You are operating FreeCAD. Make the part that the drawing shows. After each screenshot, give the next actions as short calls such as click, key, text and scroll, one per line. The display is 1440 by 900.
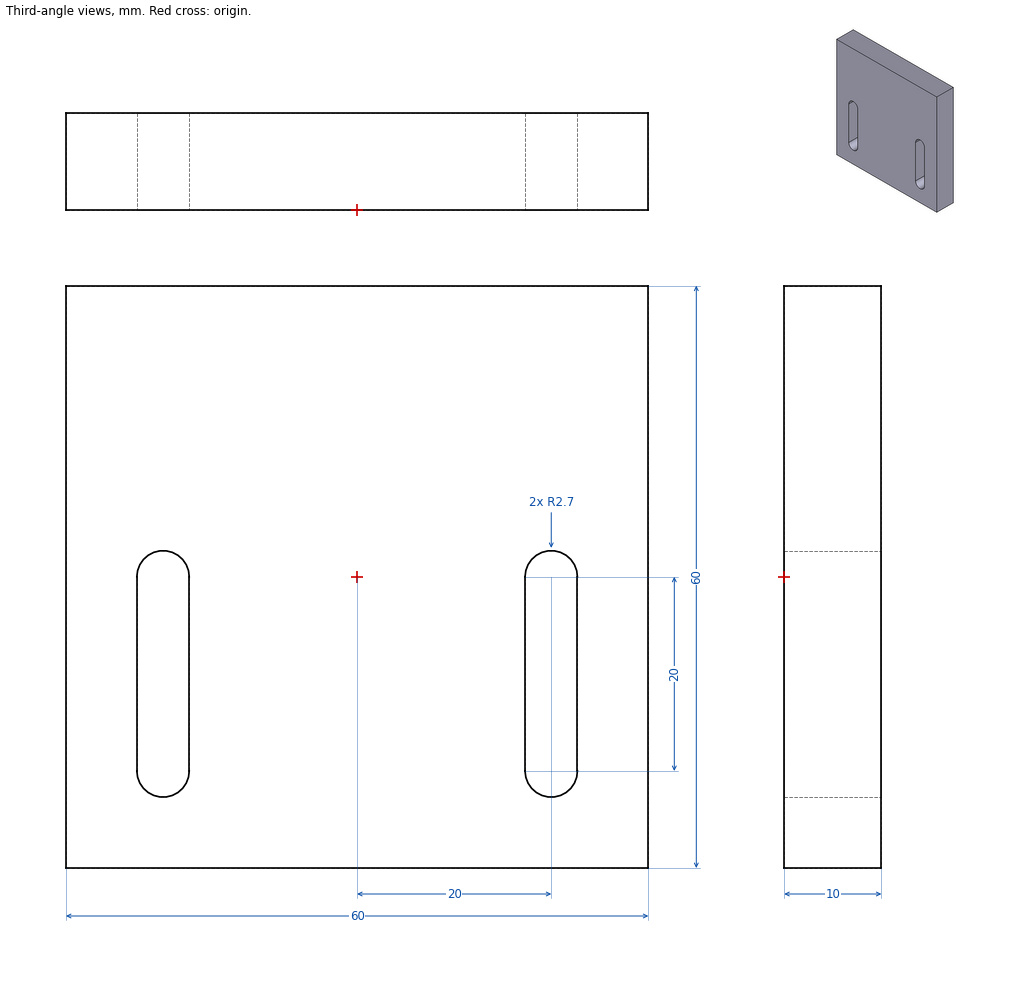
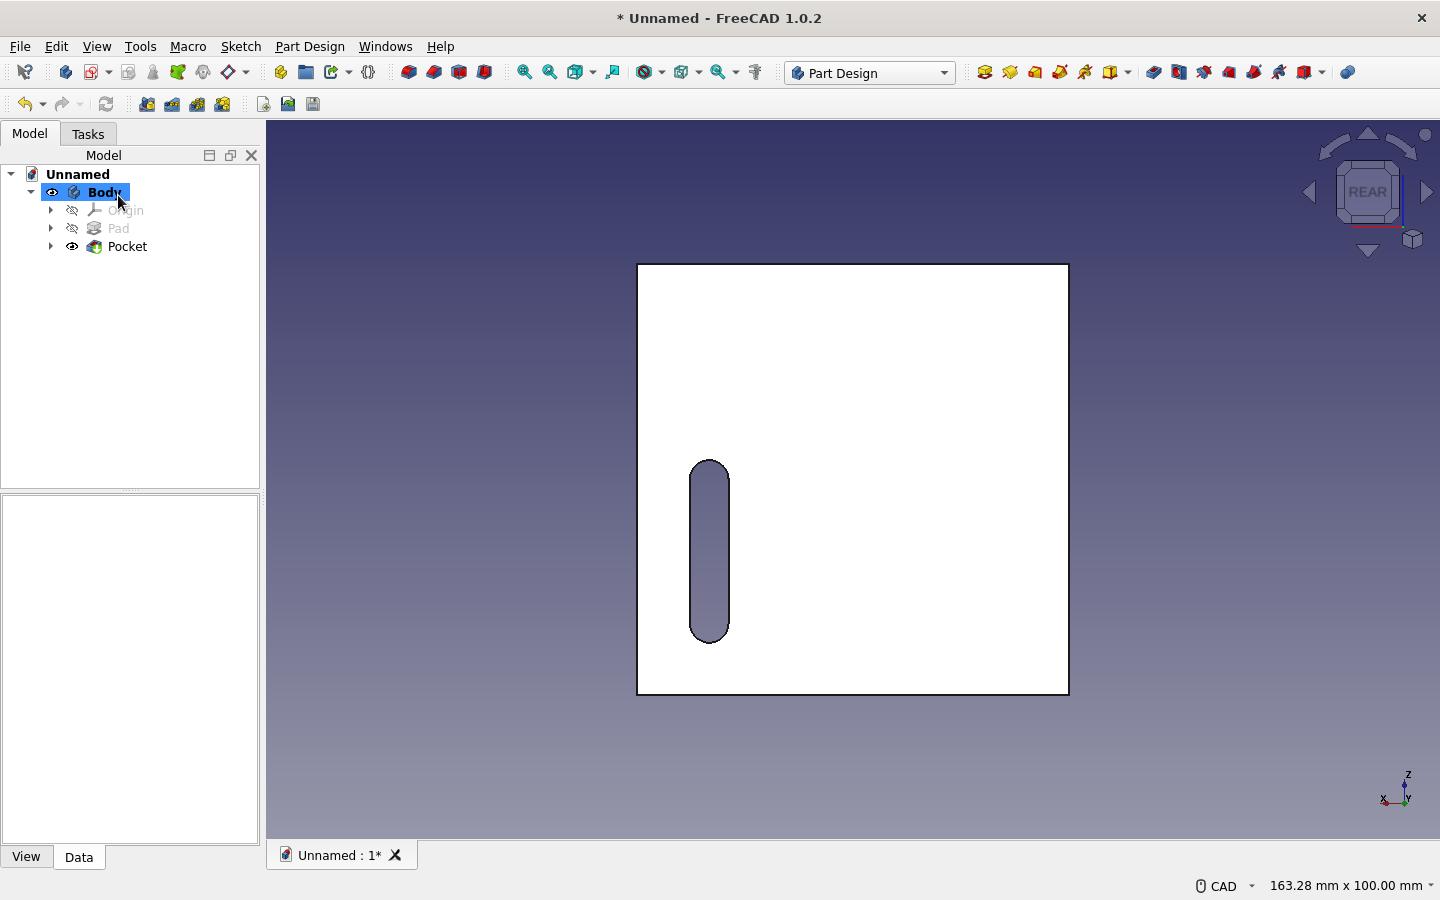
click(117, 246)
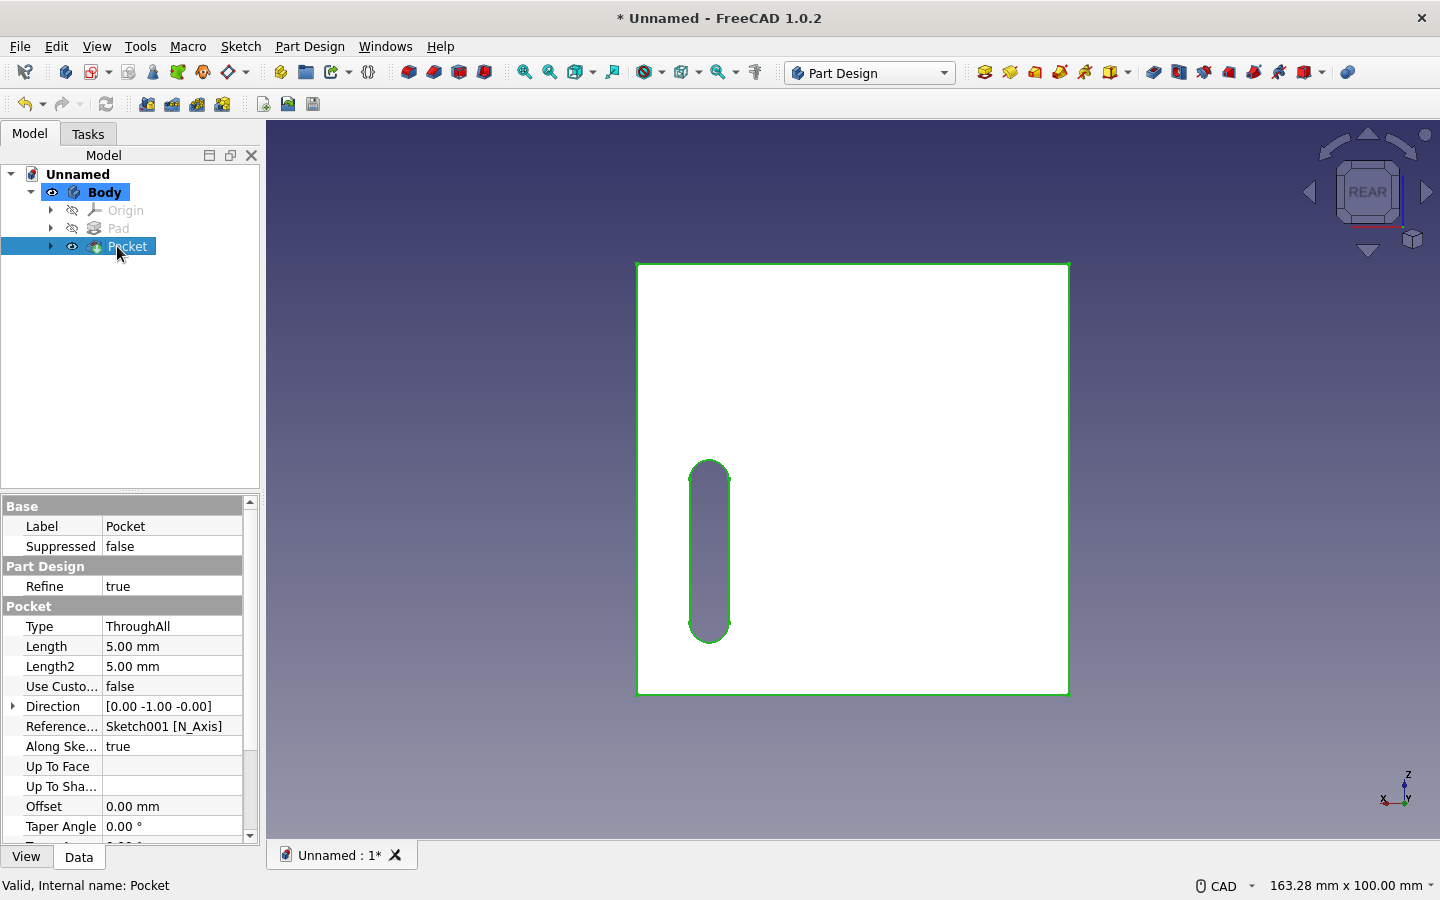
click(147, 104)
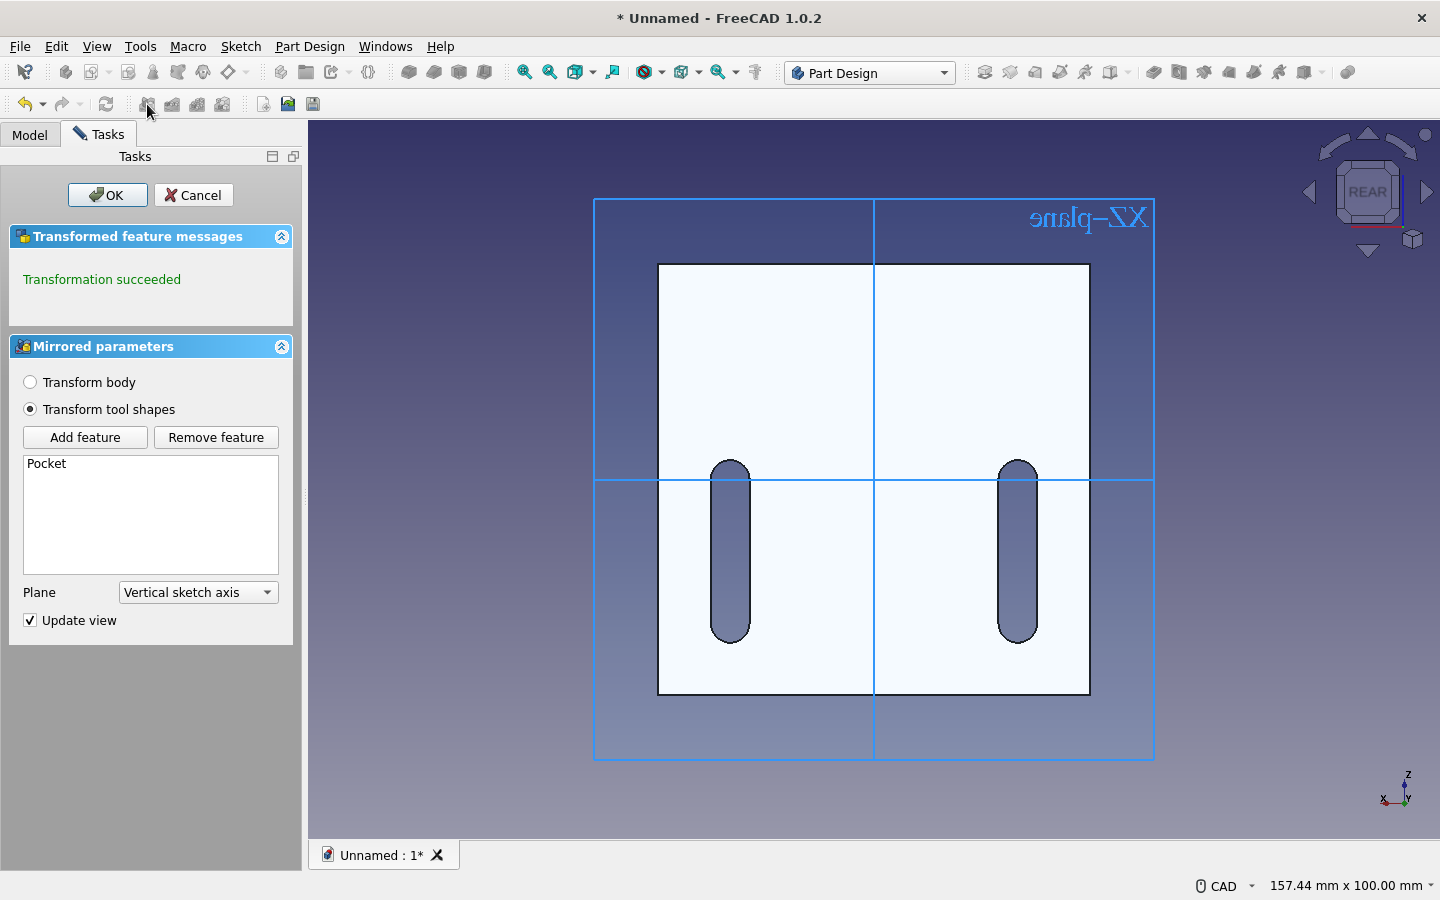
click(199, 592)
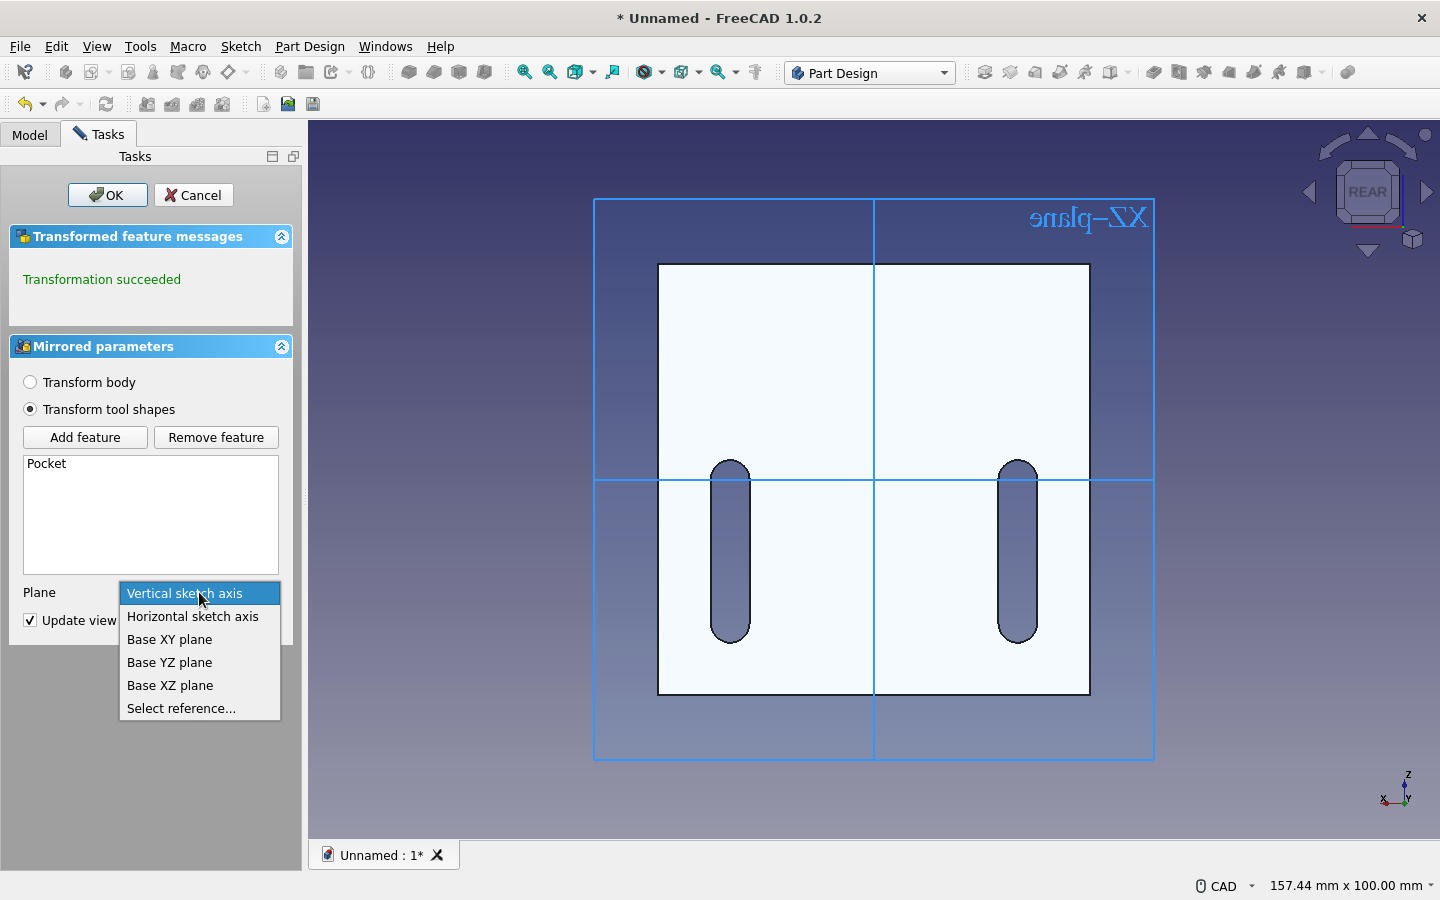
click(198, 662)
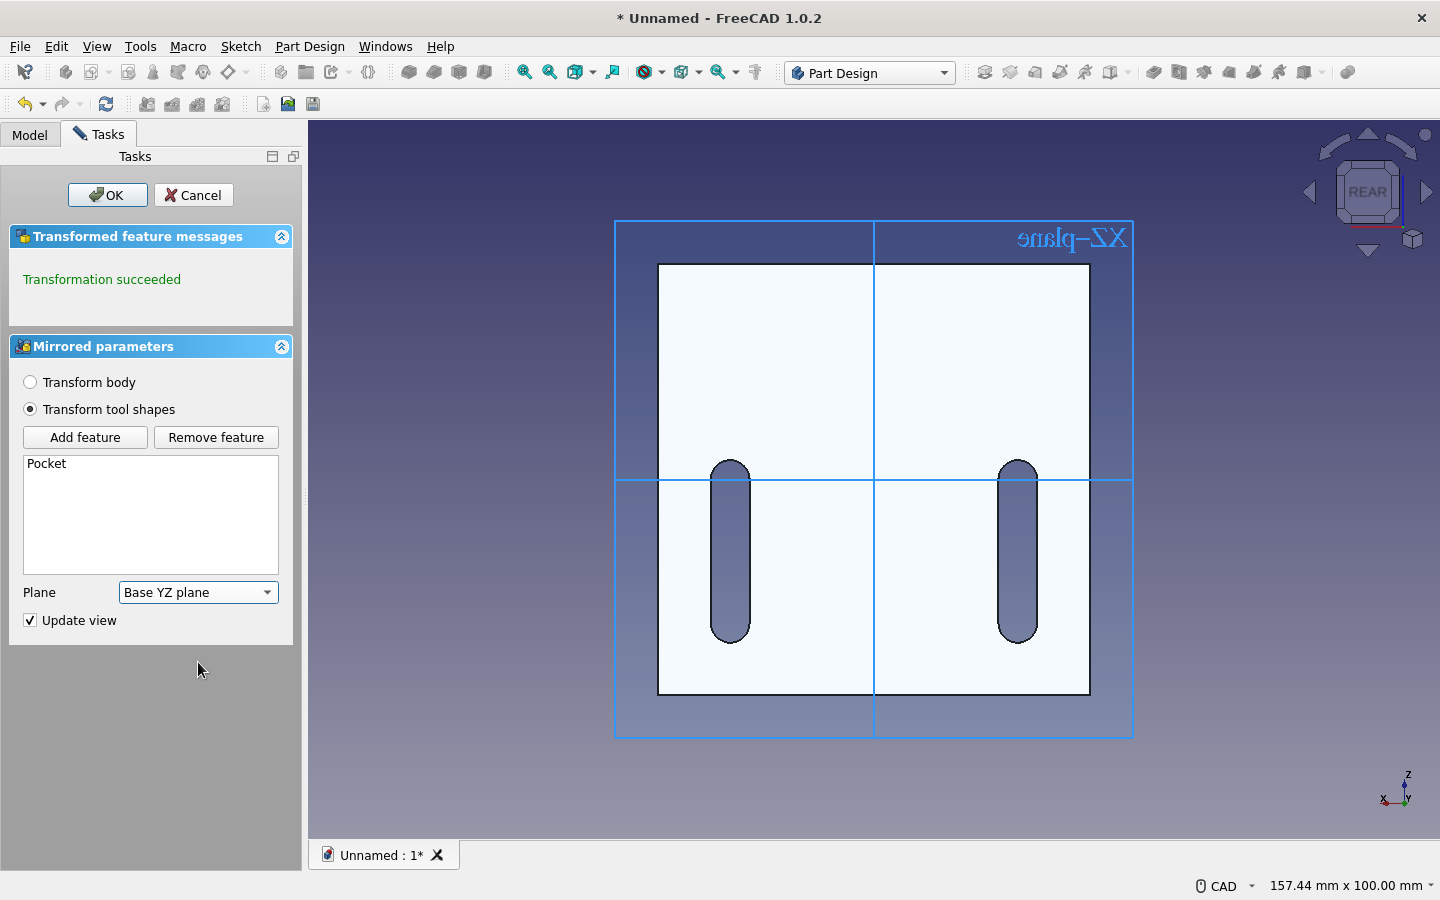
click(108, 195)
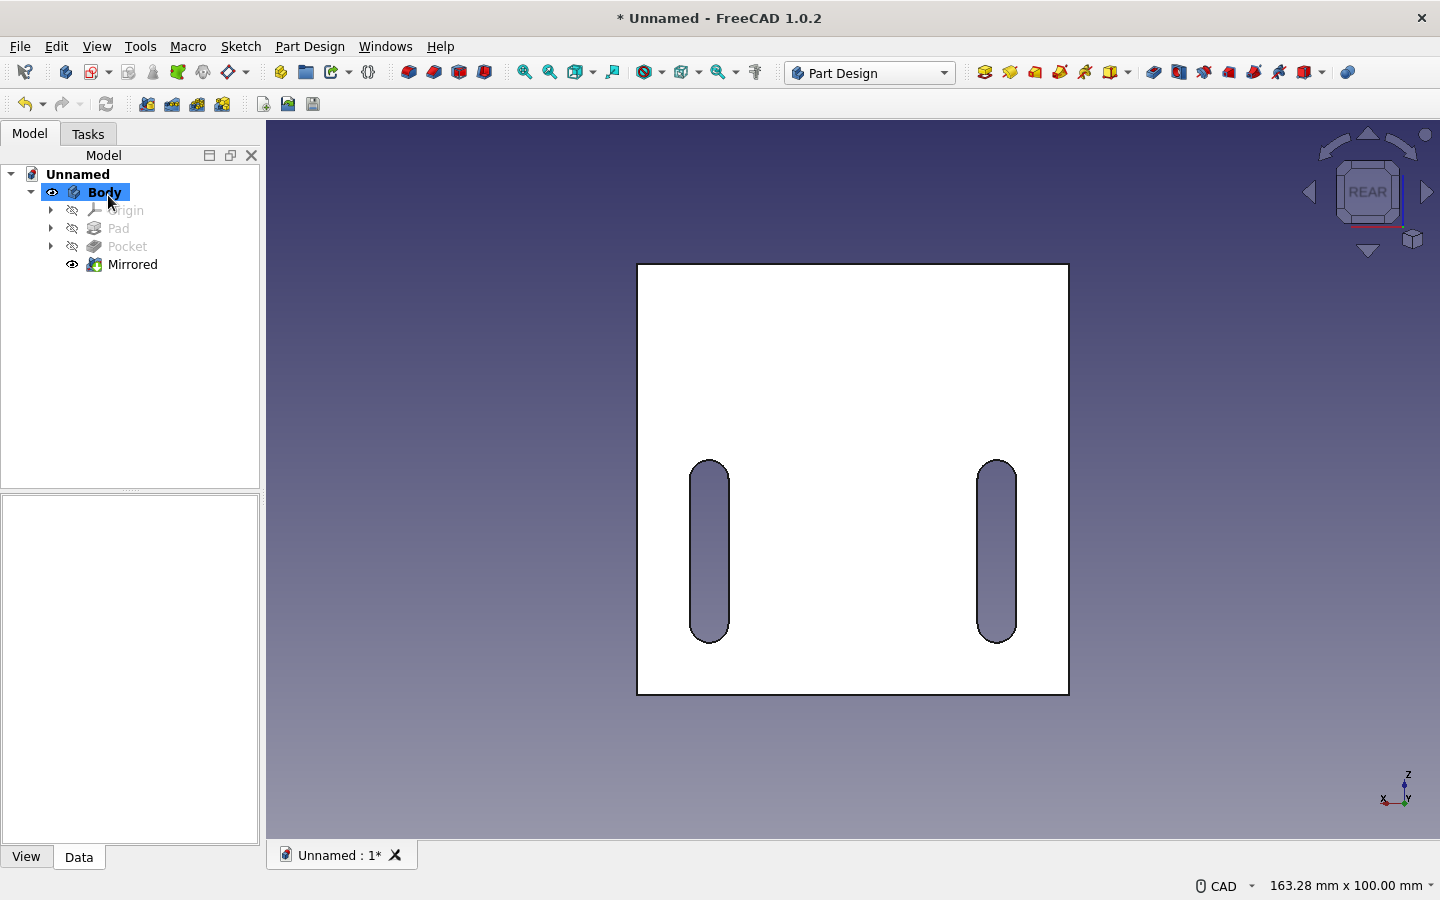
key(0)